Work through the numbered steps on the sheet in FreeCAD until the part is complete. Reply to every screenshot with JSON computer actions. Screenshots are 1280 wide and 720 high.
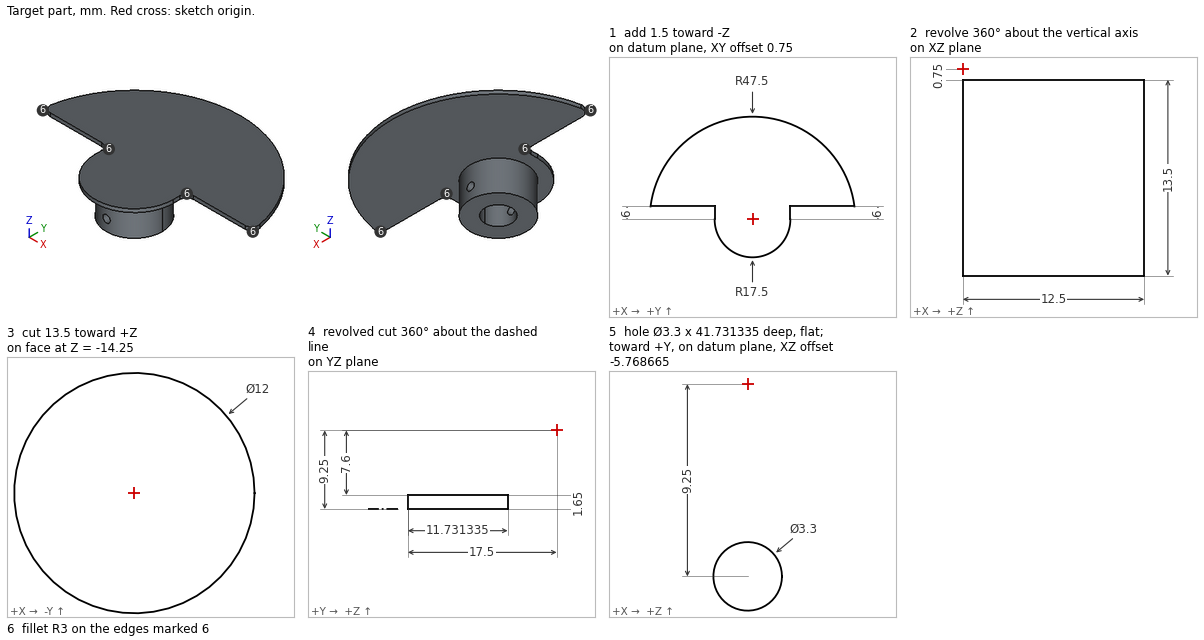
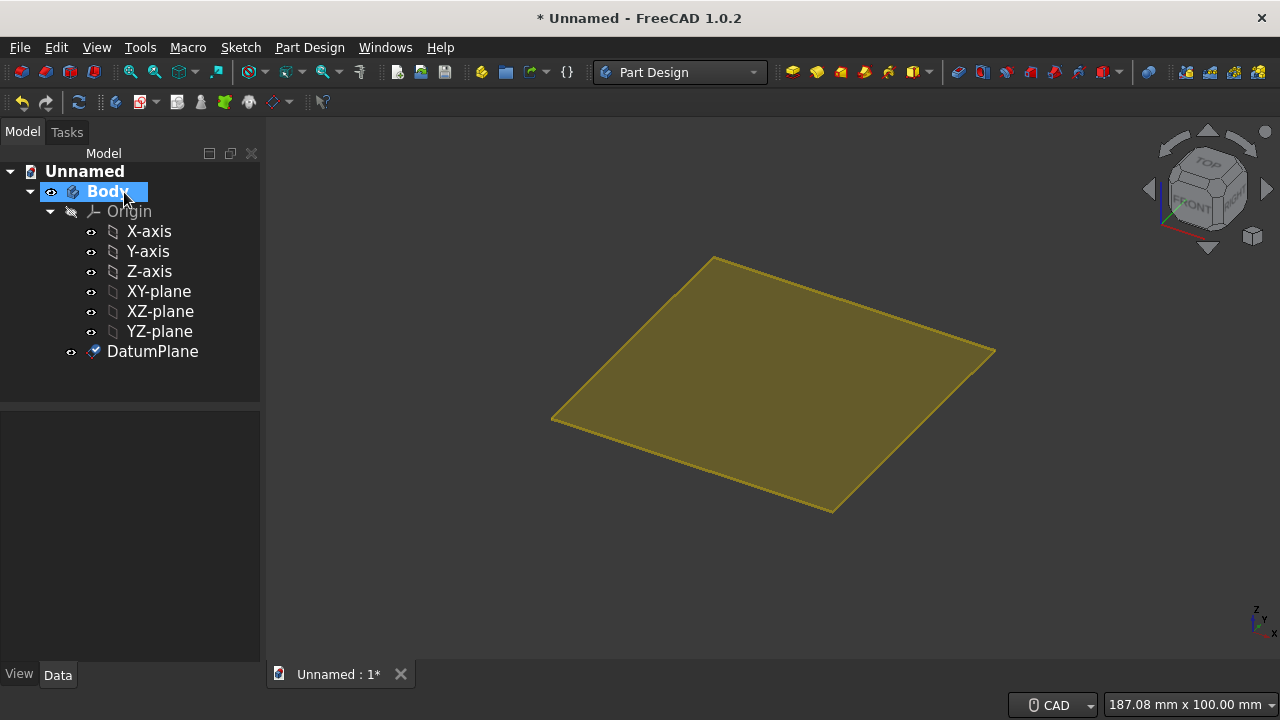
{"action": "left_click", "coordinate": [116, 352]}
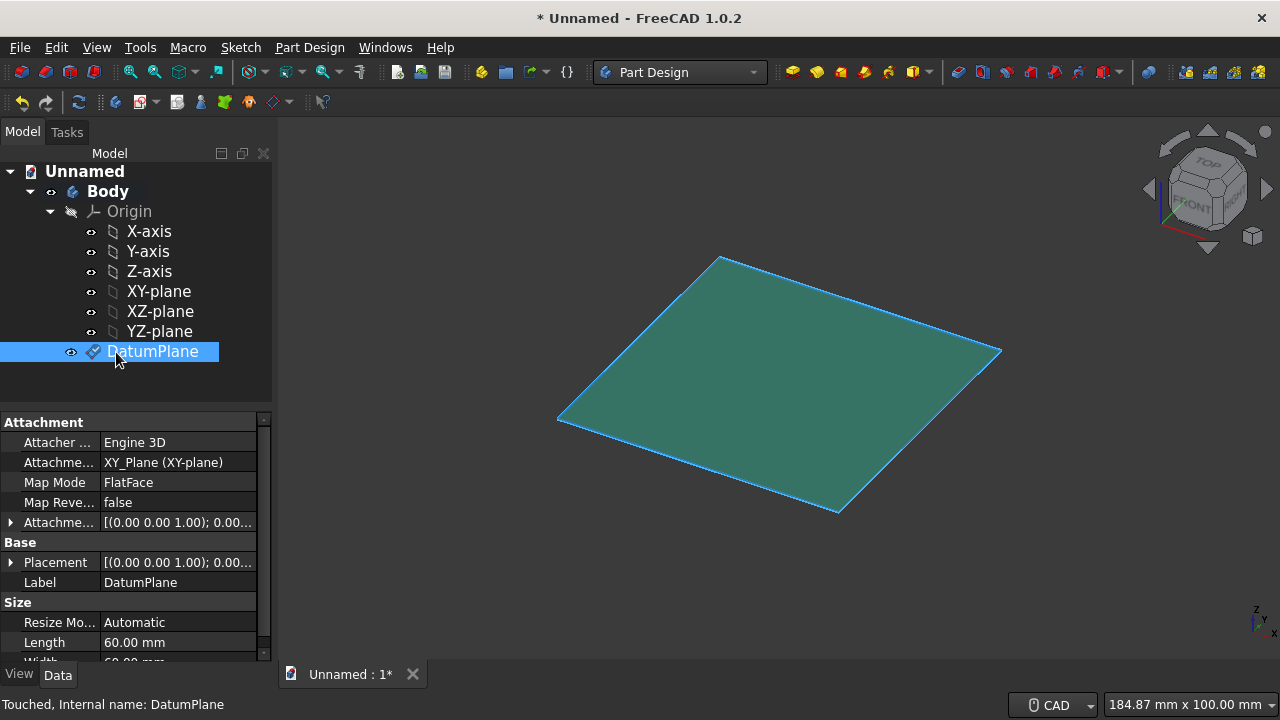
{"action": "left_click", "coordinate": [140, 102]}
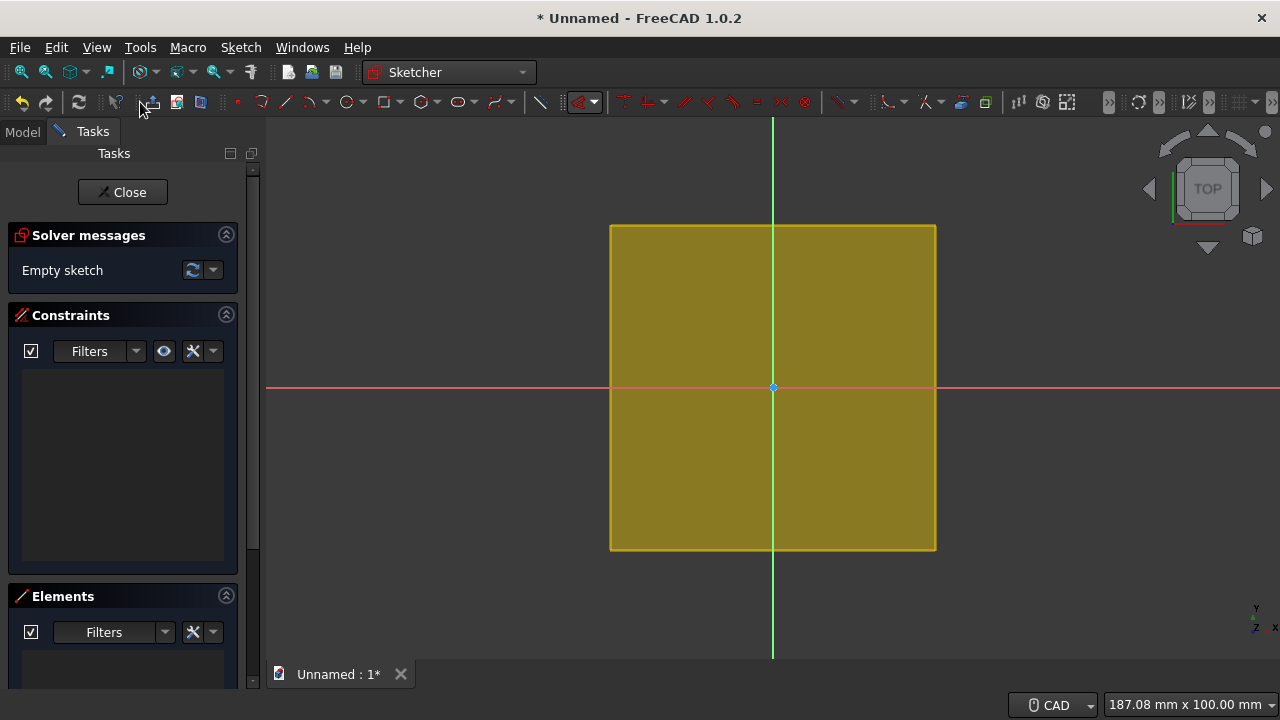
{"action": "scroll", "coordinate": [395, 631], "scroll_direction": "down", "scroll_amount": 1}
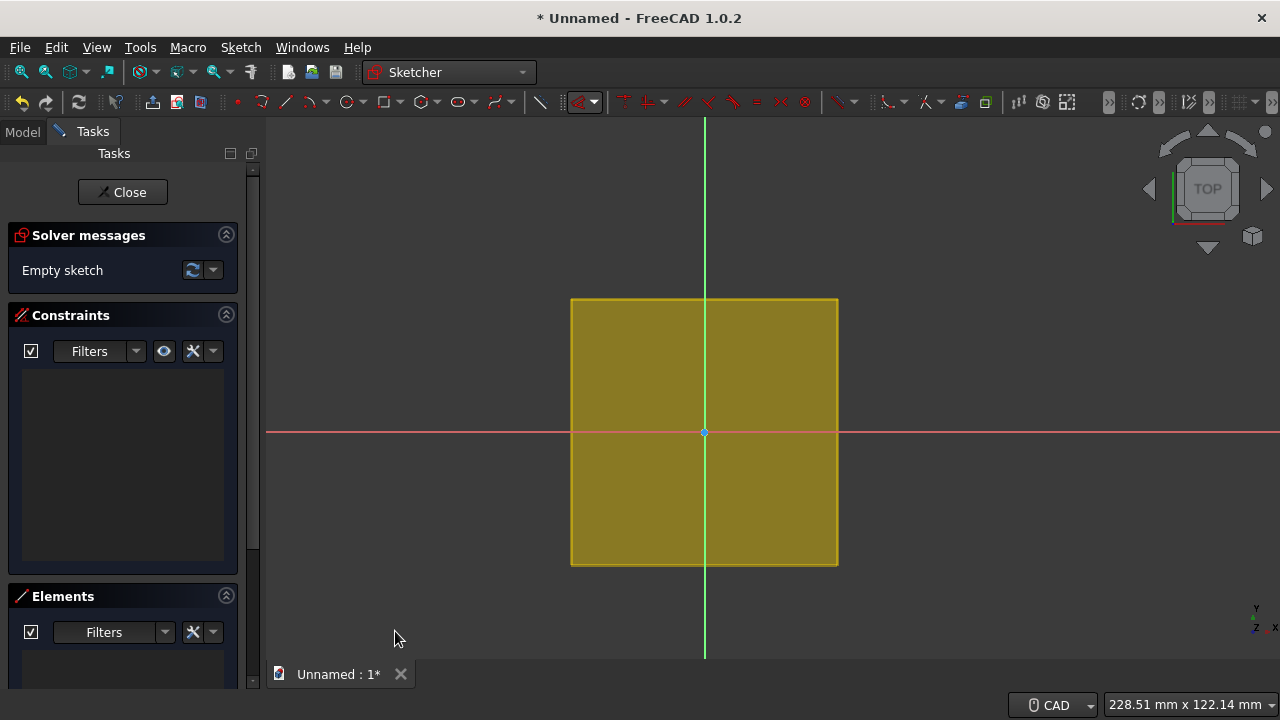
{"action": "left_click", "coordinate": [262, 102]}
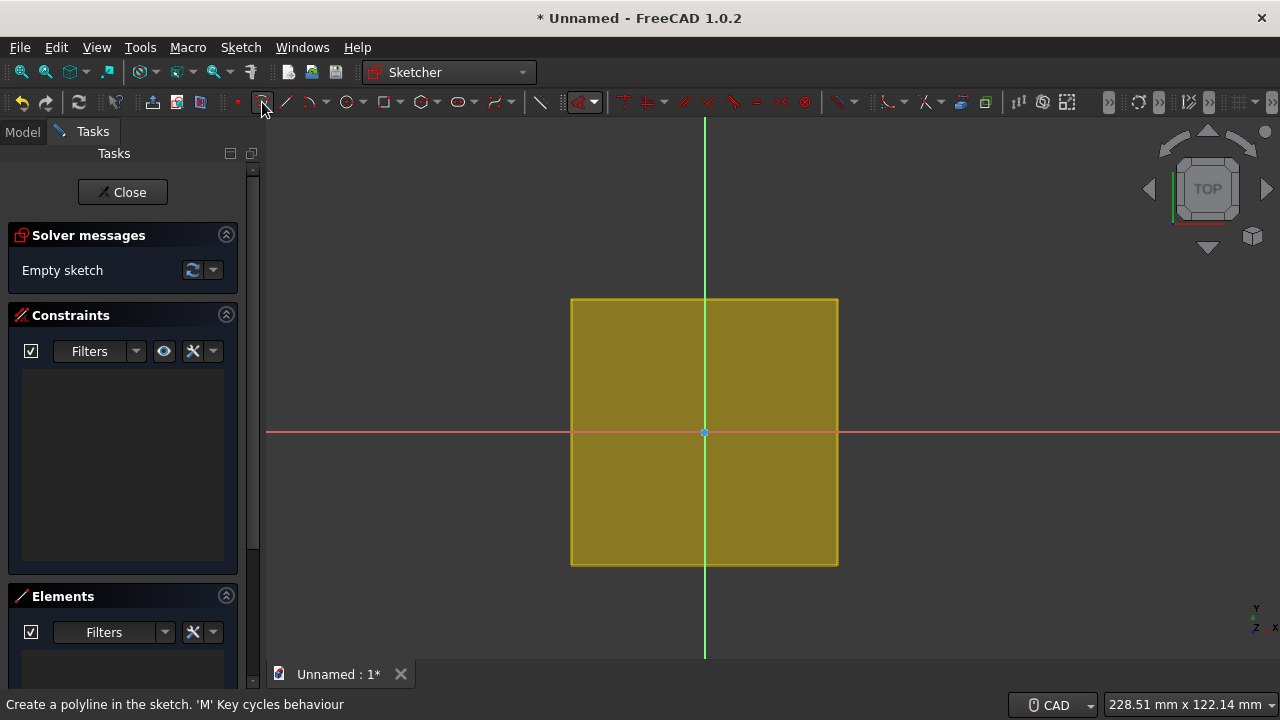
{"action": "left_click", "coordinate": [495, 406]}
{"action": "left_click", "coordinate": [627, 406]}
{"action": "left_click", "coordinate": [627, 432]}
{"action": "right_click", "coordinate": [627, 432]}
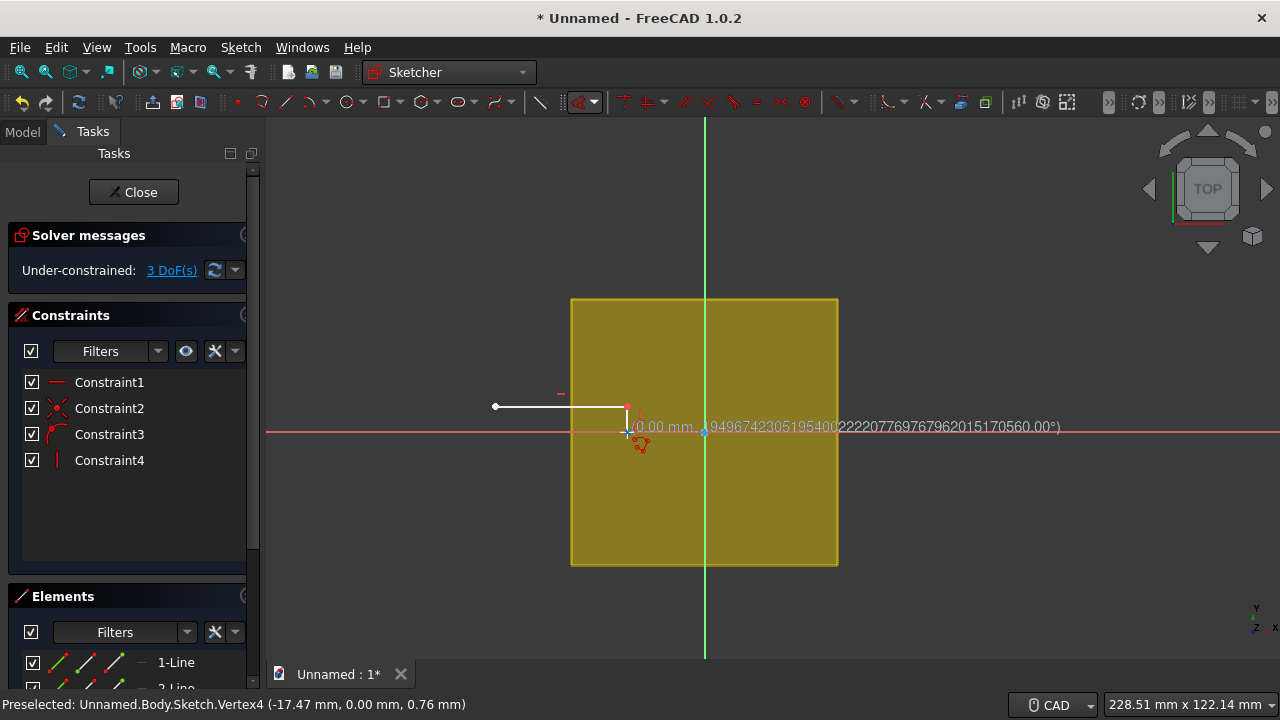
{"action": "left_click", "coordinate": [782, 432]}
{"action": "left_click", "coordinate": [782, 406]}
{"action": "left_click", "coordinate": [914, 406]}
{"action": "right_click", "coordinate": [914, 406]}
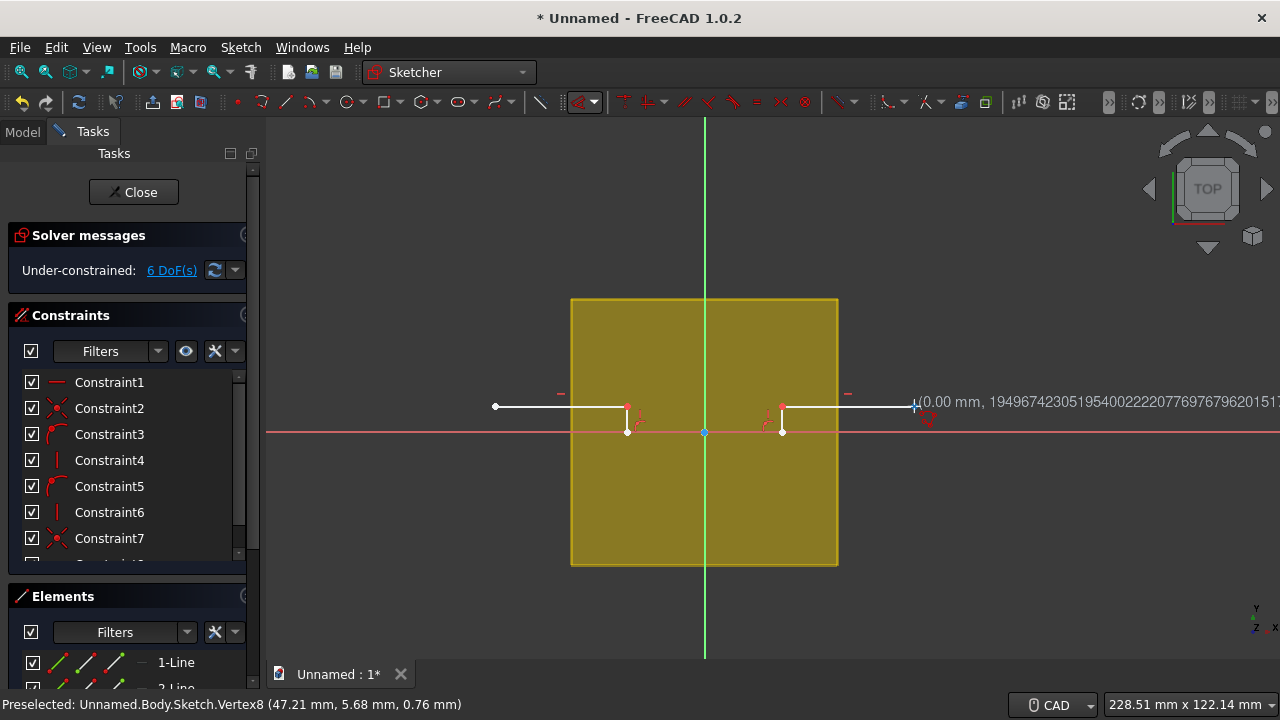
{"action": "key", "text": "g 3 a"}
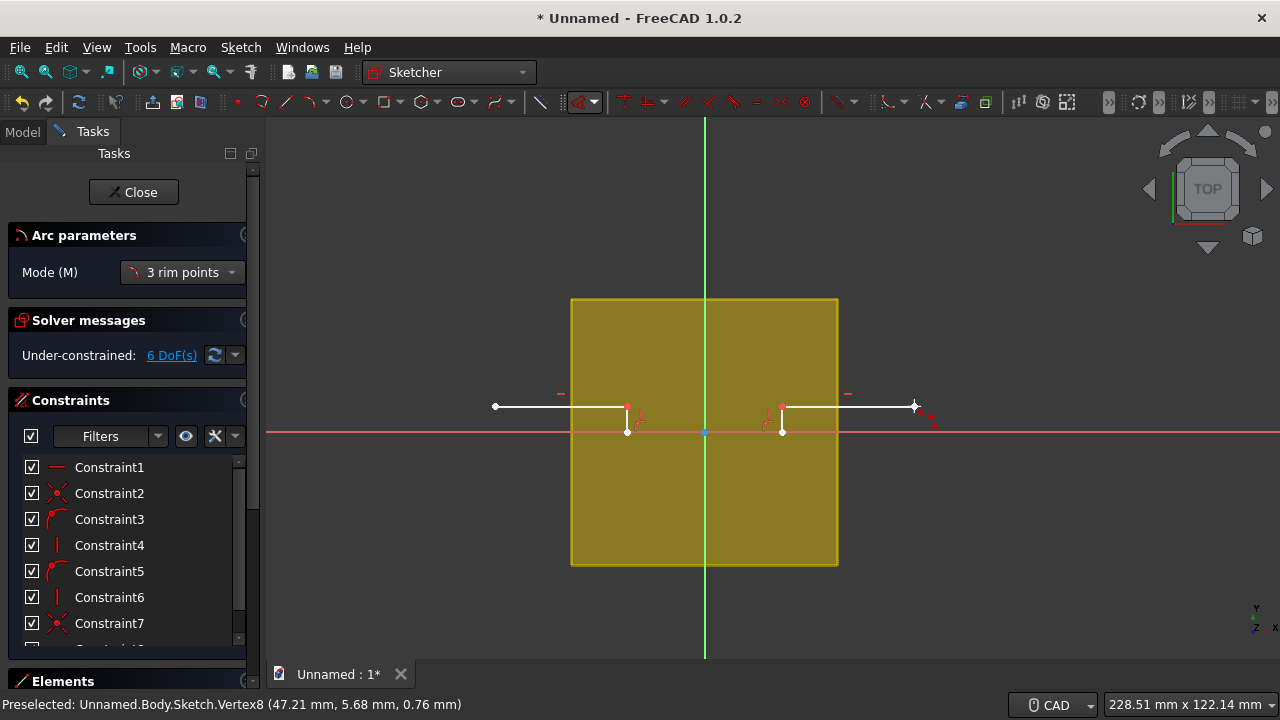
{"action": "left_click", "coordinate": [627, 432]}
{"action": "left_click", "coordinate": [782, 432]}
{"action": "left_click", "coordinate": [681, 506]}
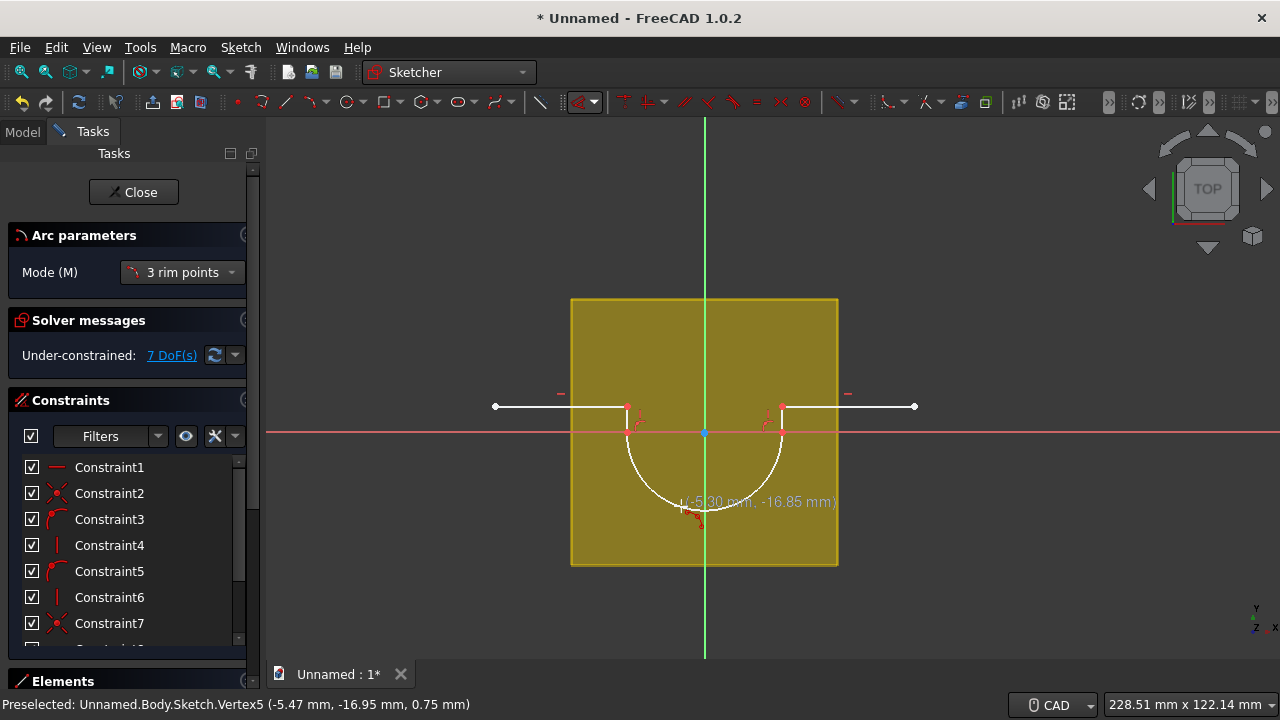
{"action": "left_click", "coordinate": [914, 407]}
{"action": "left_click", "coordinate": [495, 407]}
{"action": "left_click", "coordinate": [765, 230]}
{"action": "key", "text": "Escape"}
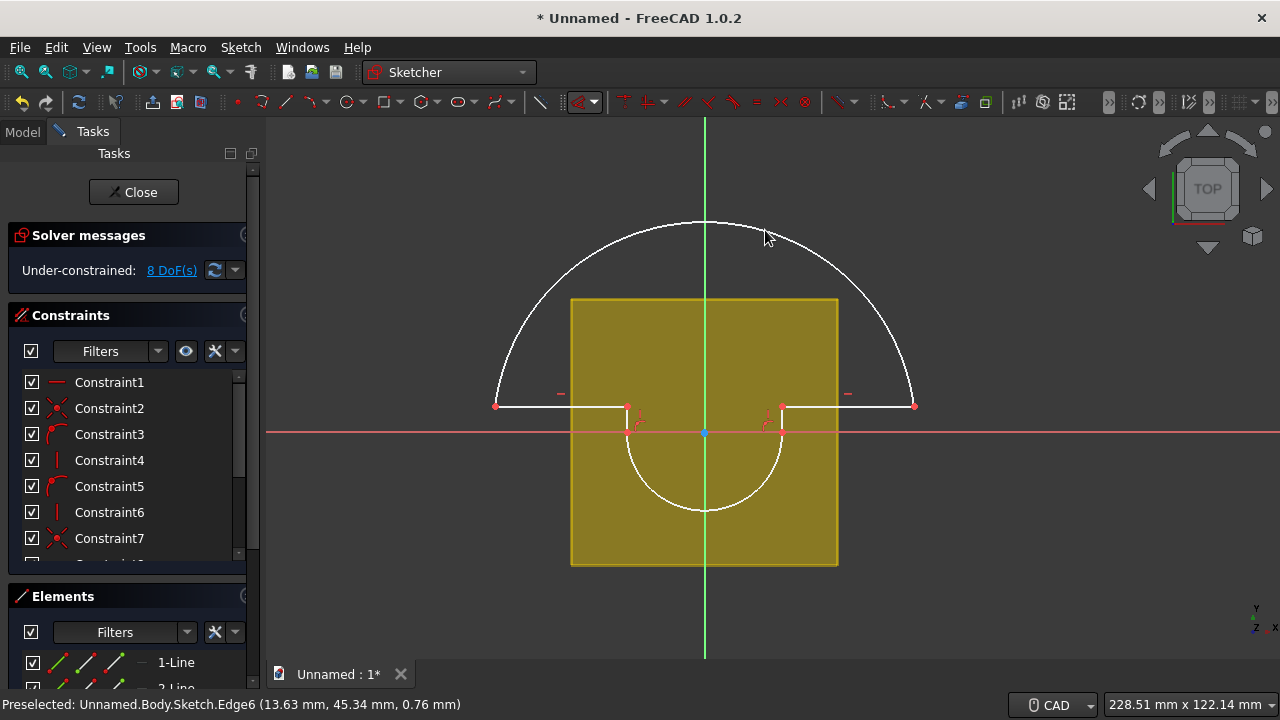
{"action": "scroll", "coordinate": [627, 417], "scroll_direction": "up", "scroll_amount": 2}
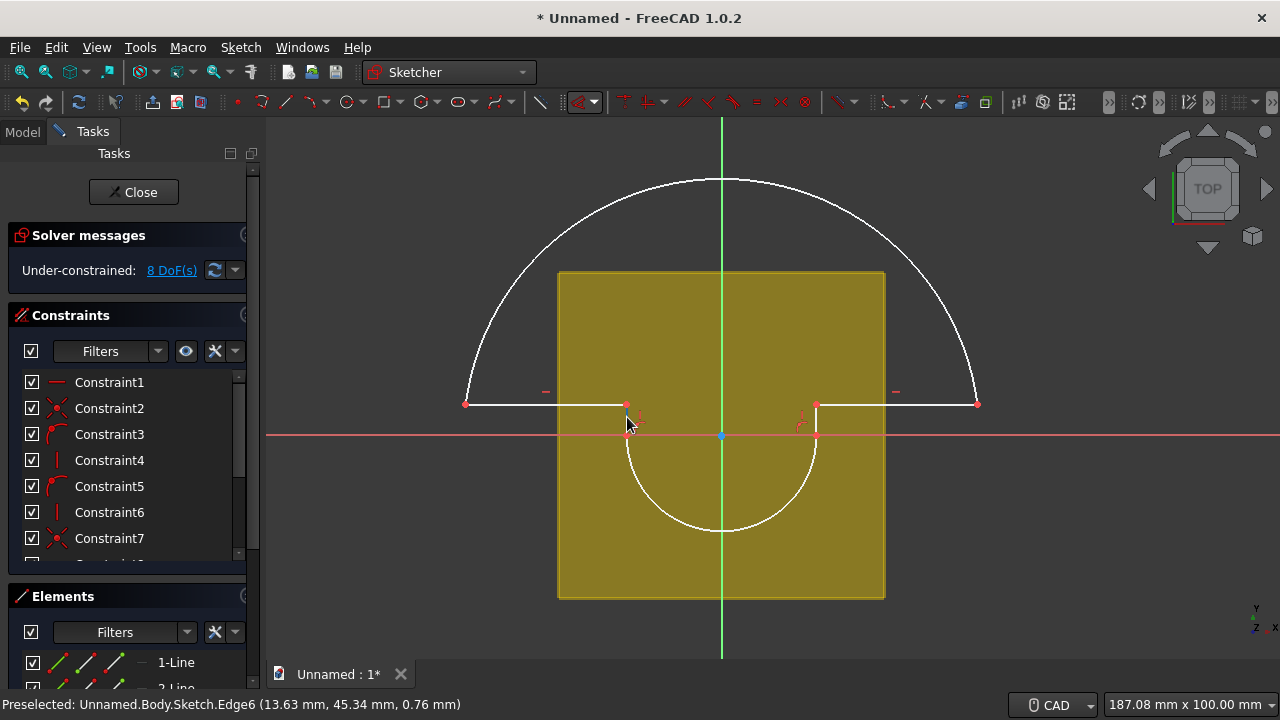
{"action": "left_click", "coordinate": [627, 417]}